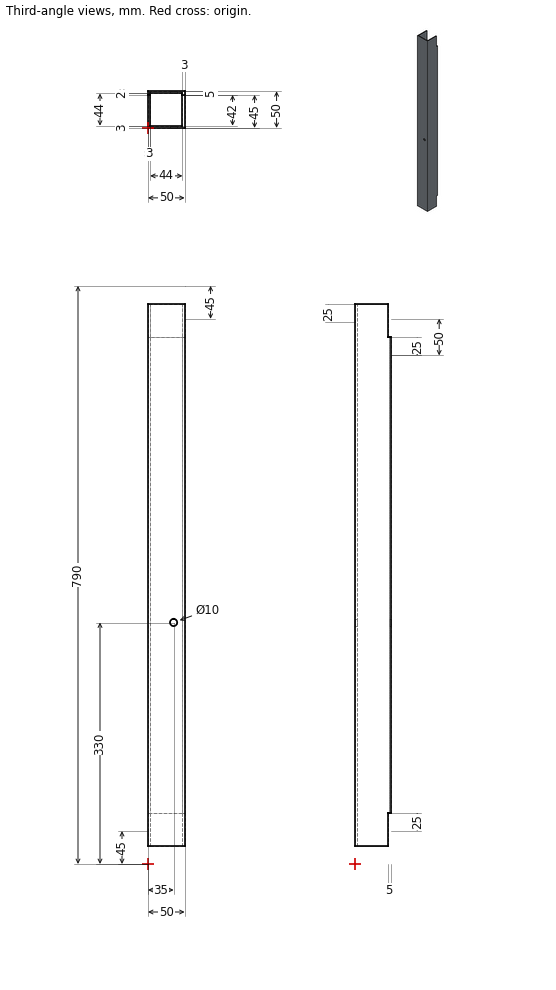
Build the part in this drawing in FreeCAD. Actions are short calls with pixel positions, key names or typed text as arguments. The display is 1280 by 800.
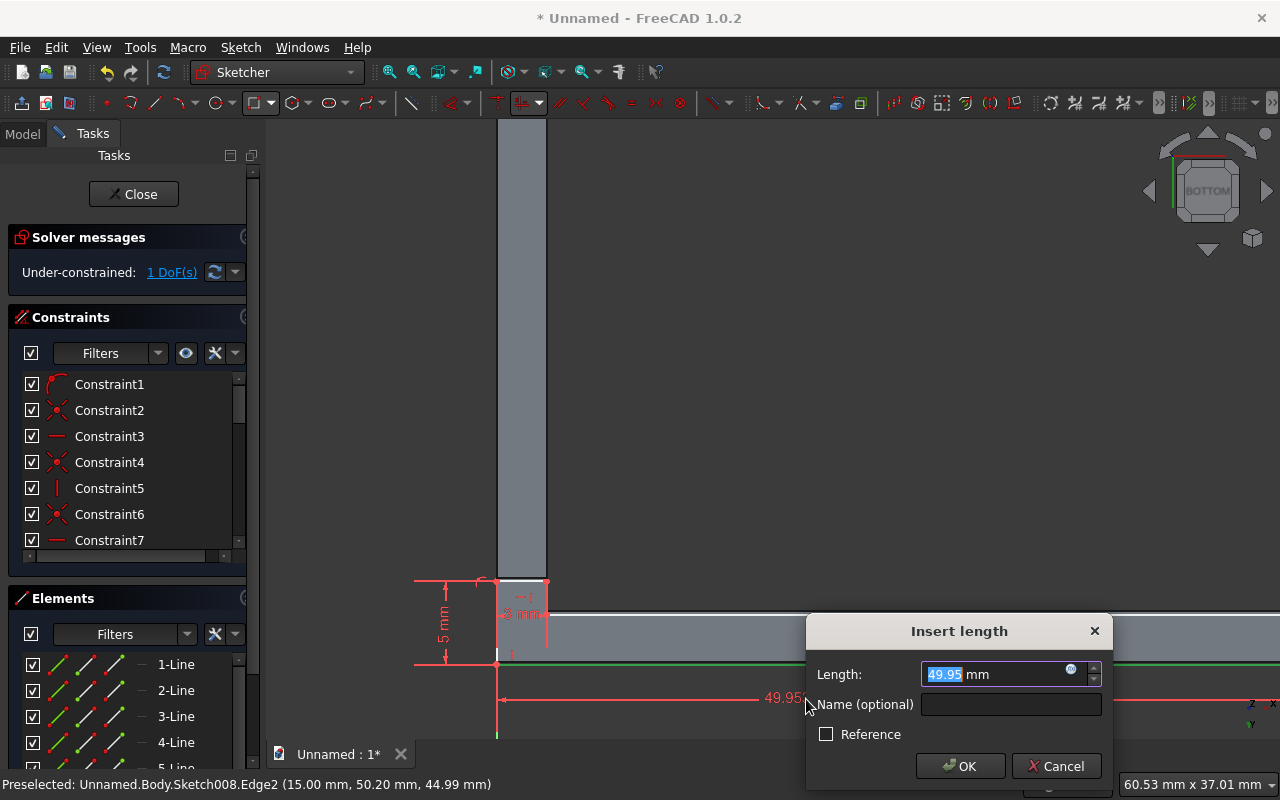
text(50)
key(Return)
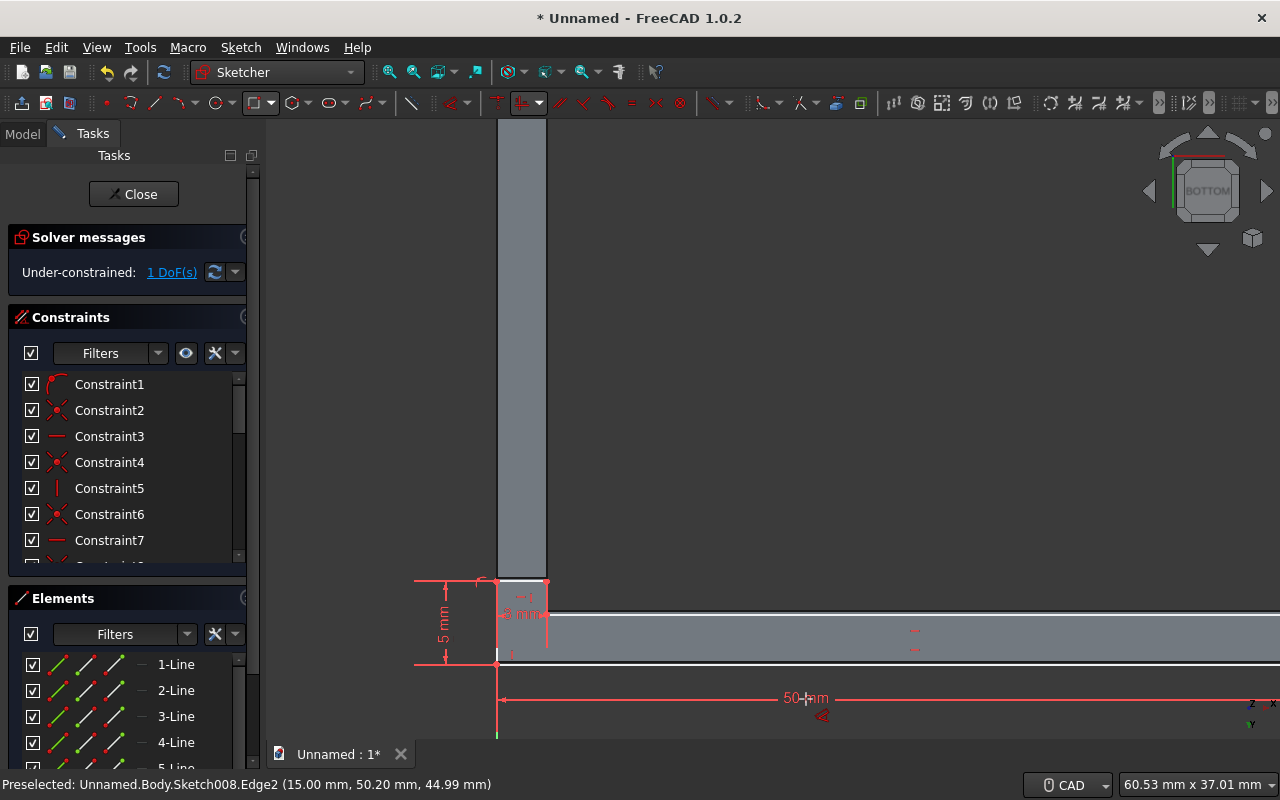
click(497, 581)
click(463, 364)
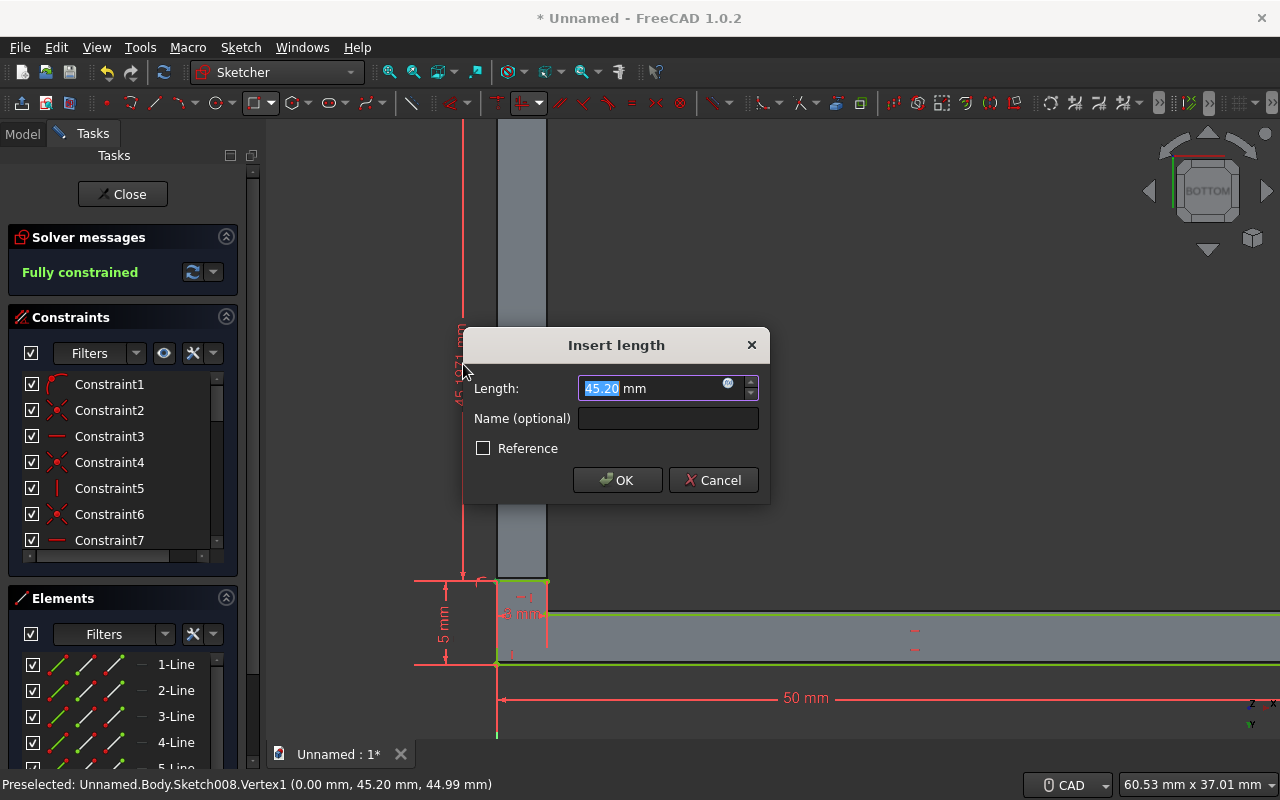
text(45)
key(Return)
key(Escape)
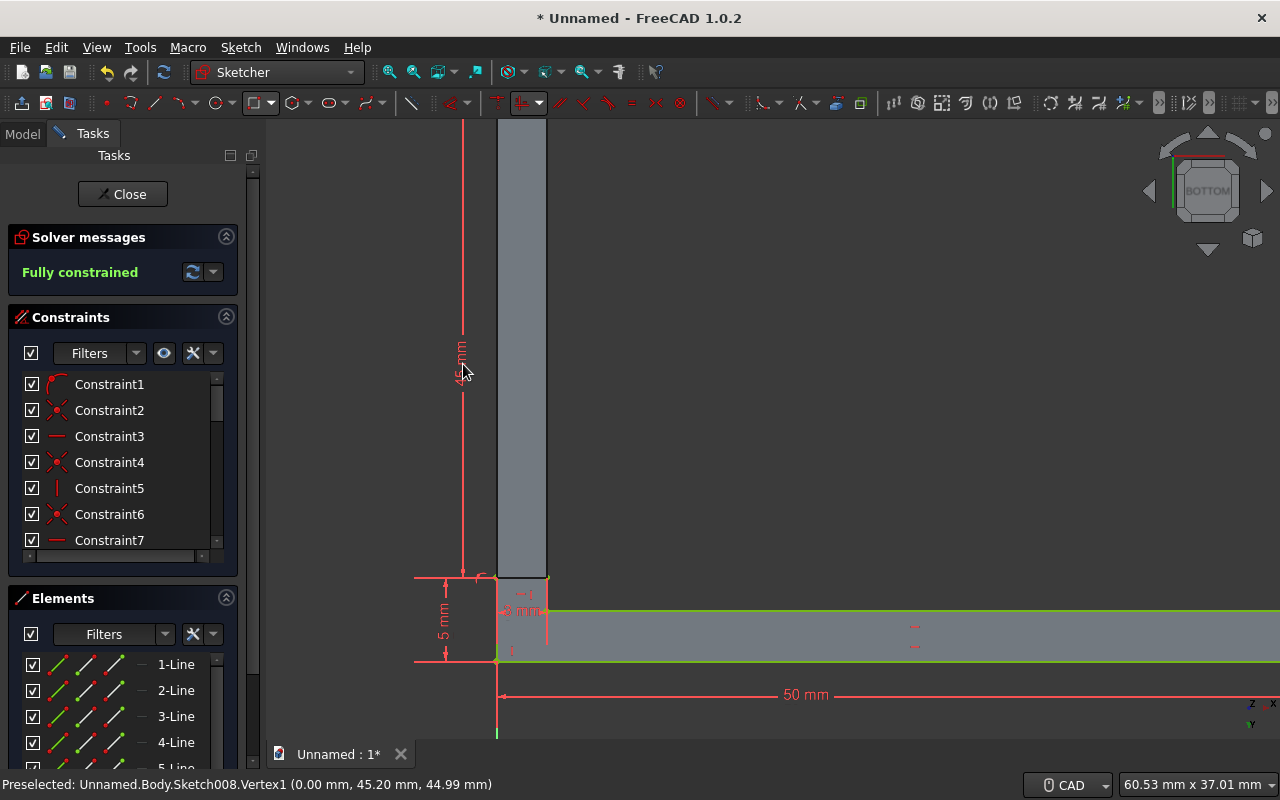
click(123, 194)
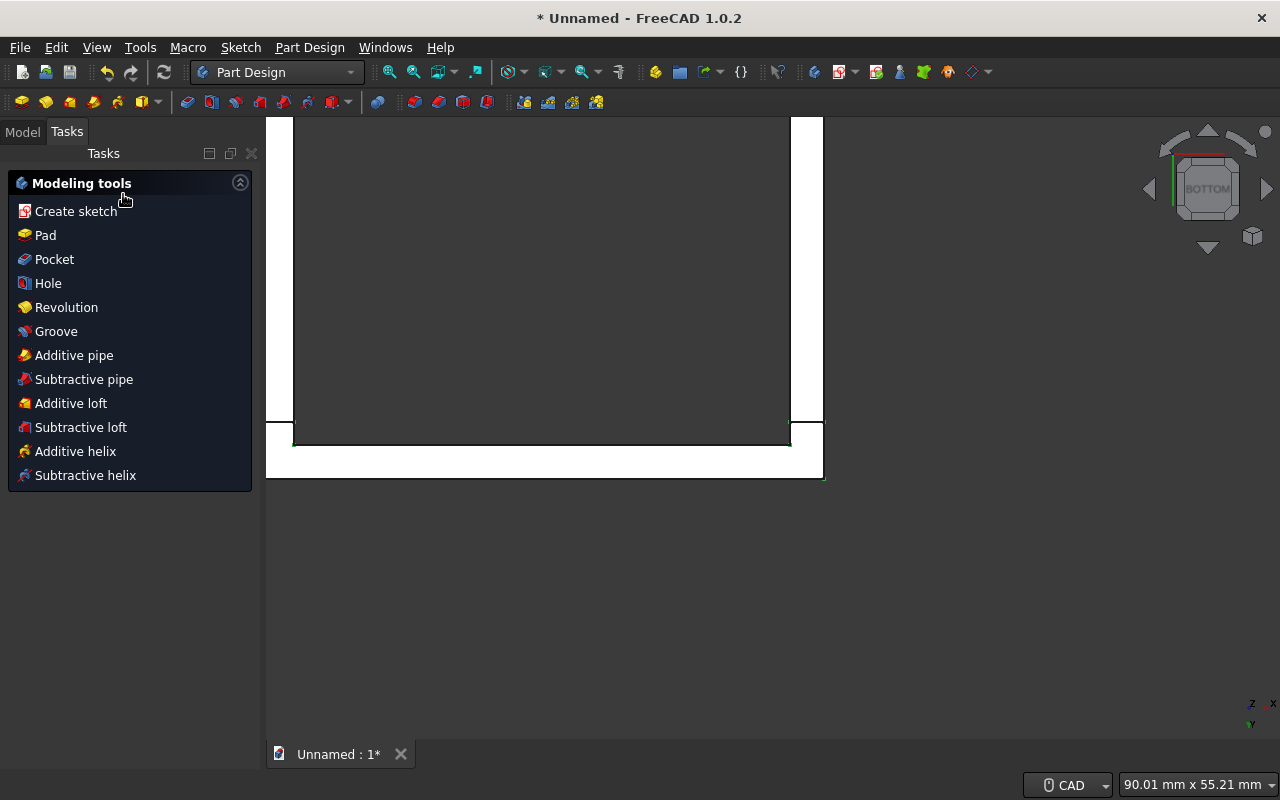
click(188, 102)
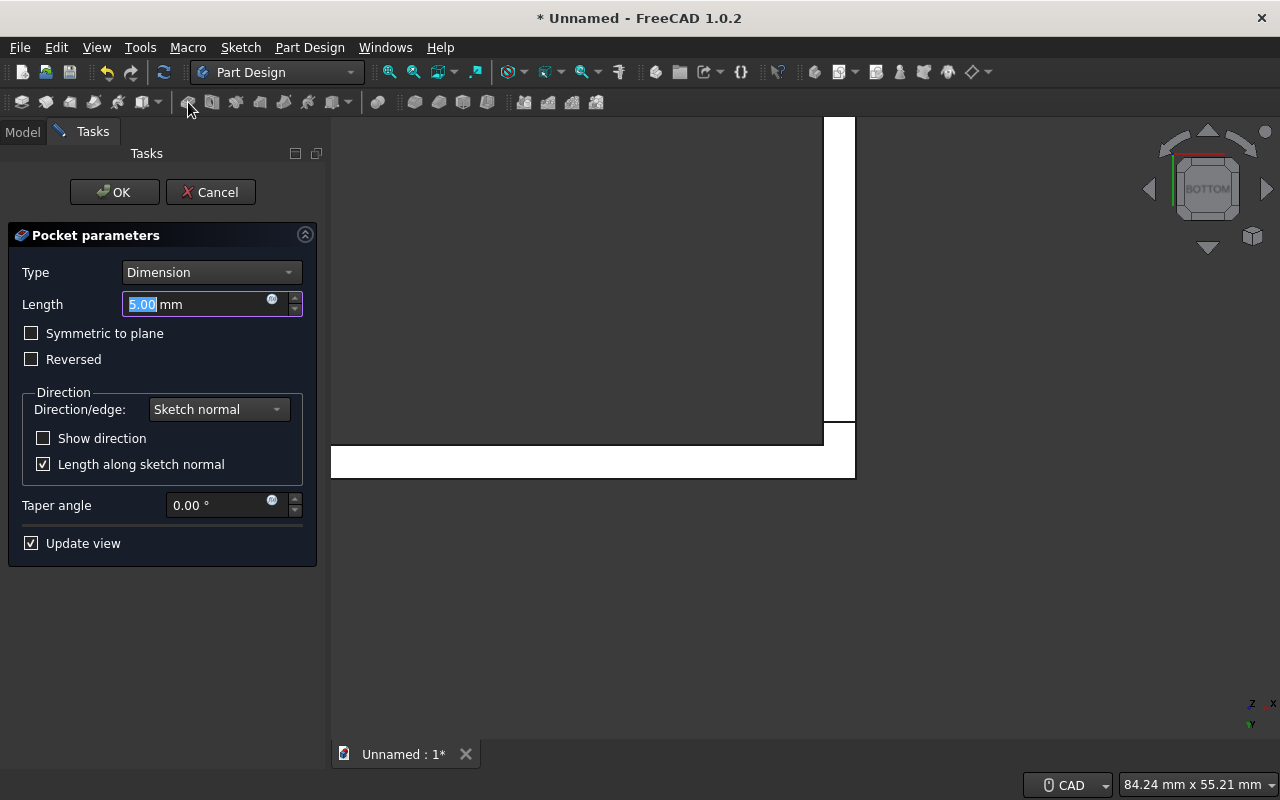
text(25)
key(Tab)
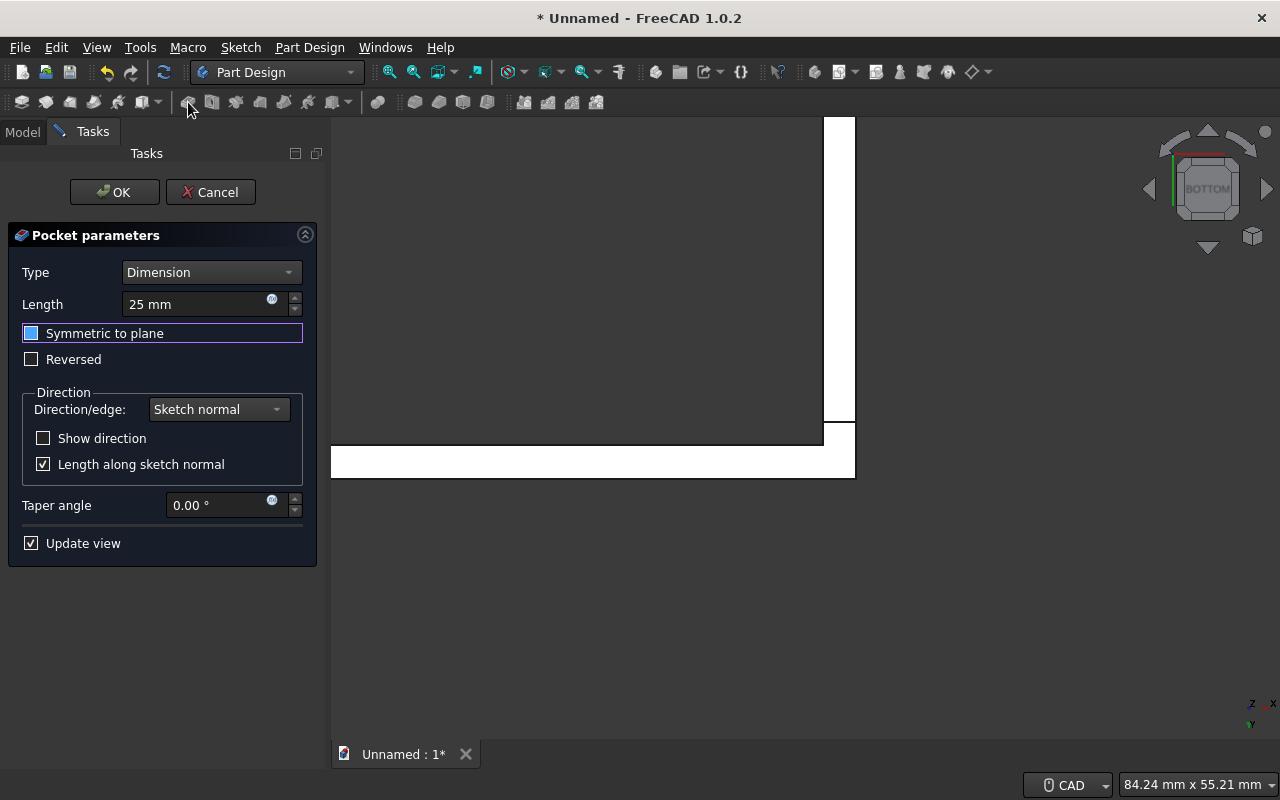
click(115, 192)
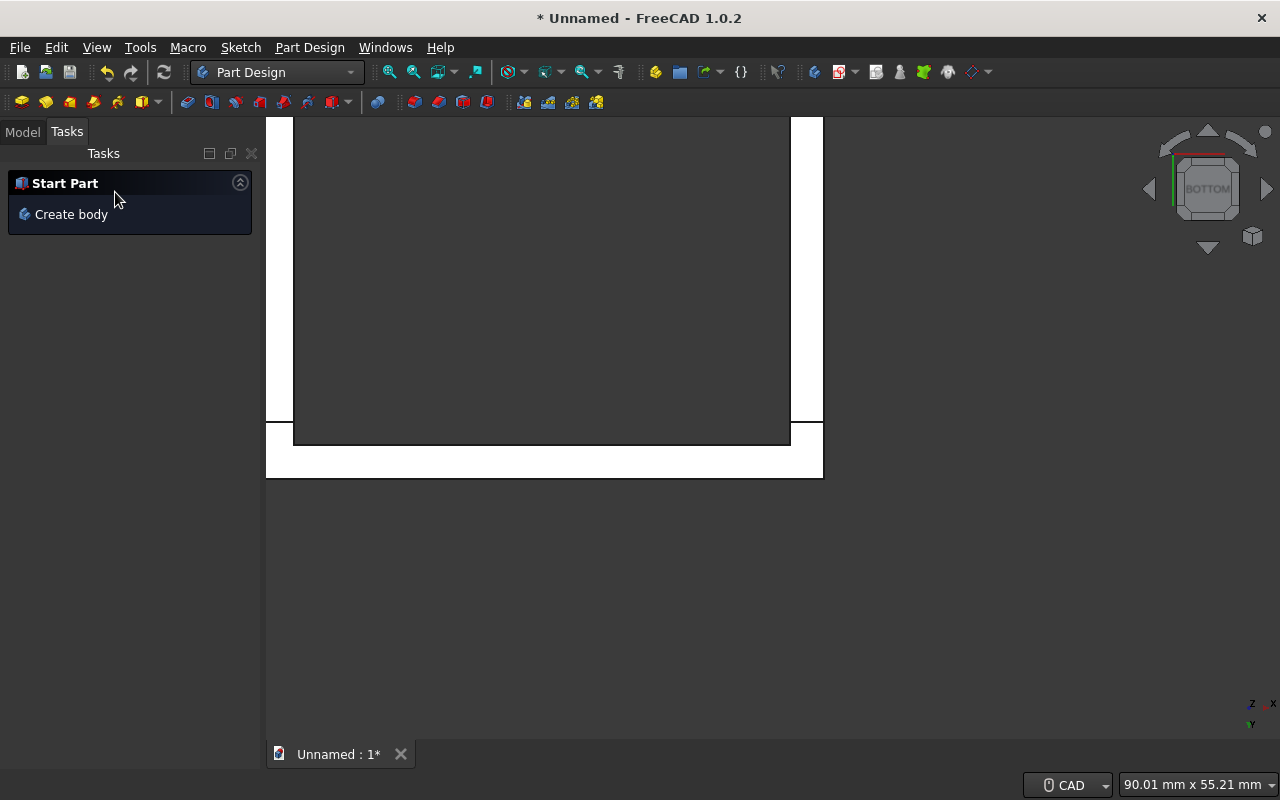
click(390, 72)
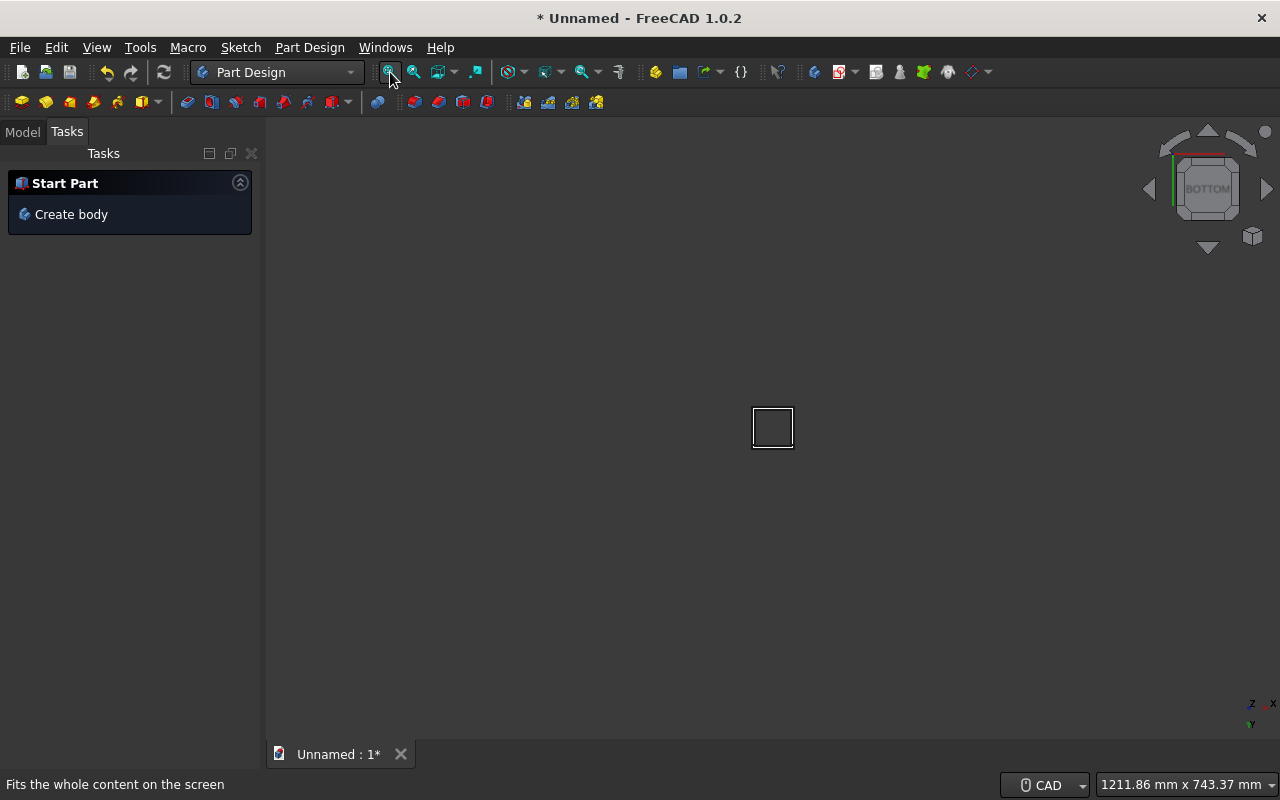
key(4)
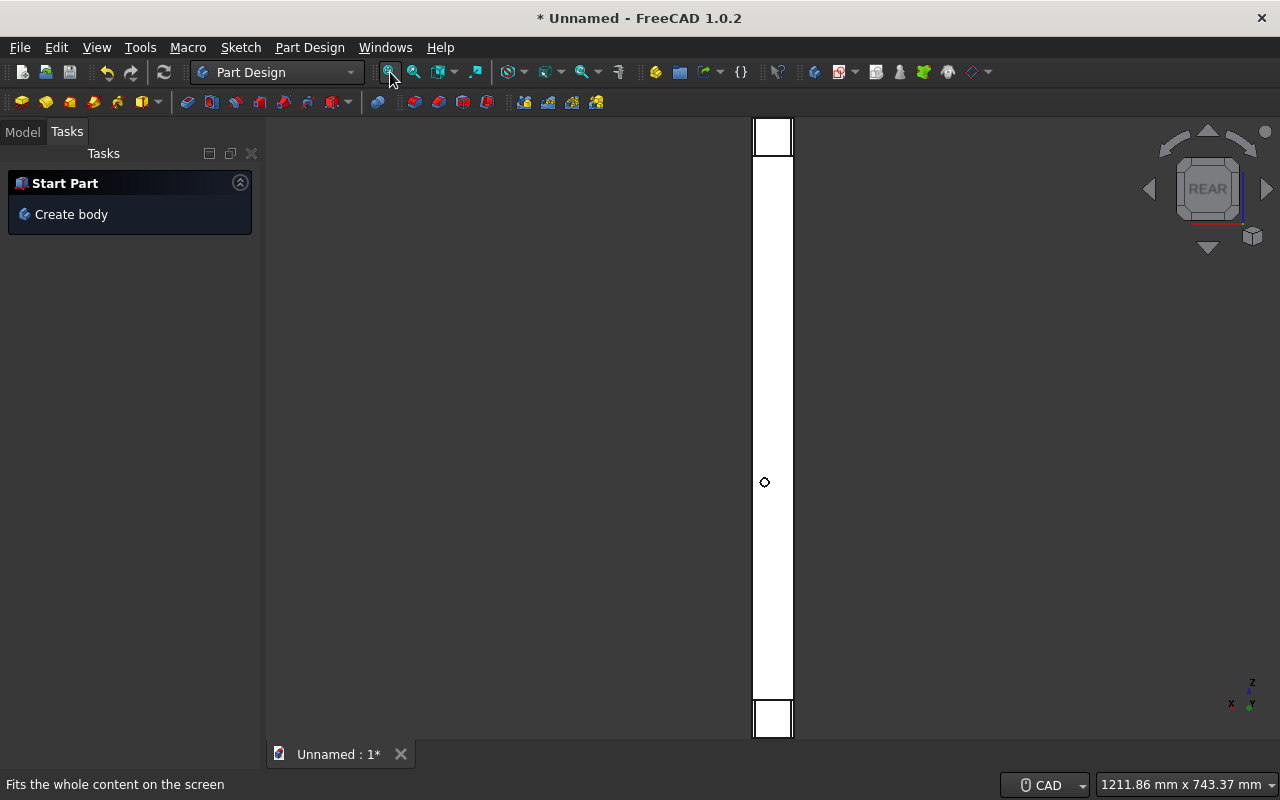
click(773, 194)